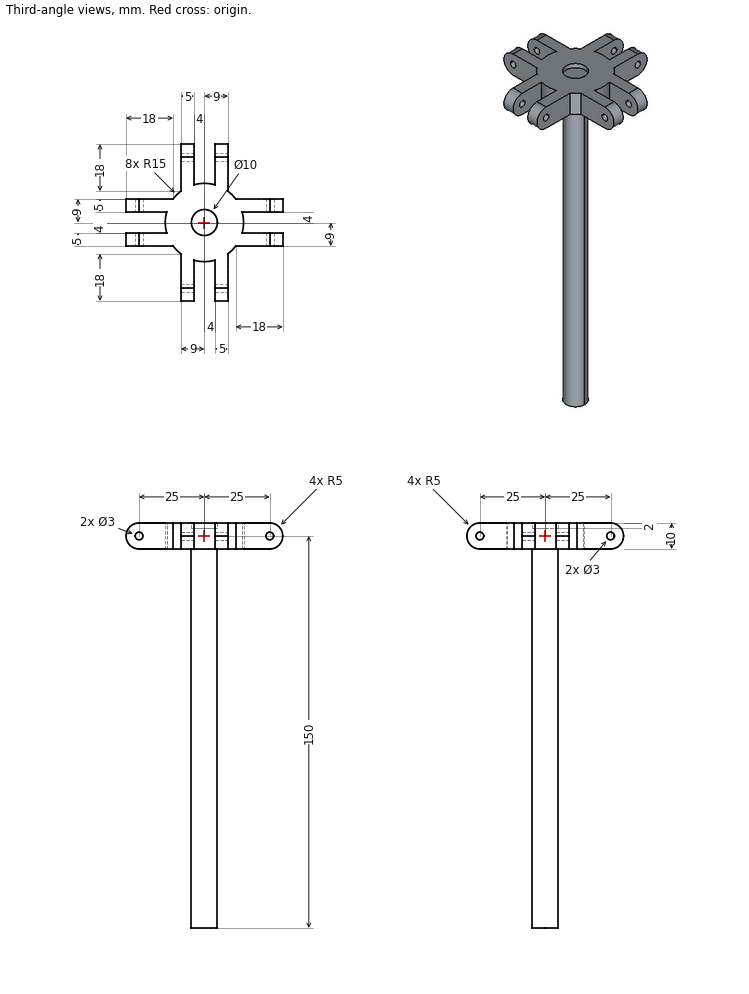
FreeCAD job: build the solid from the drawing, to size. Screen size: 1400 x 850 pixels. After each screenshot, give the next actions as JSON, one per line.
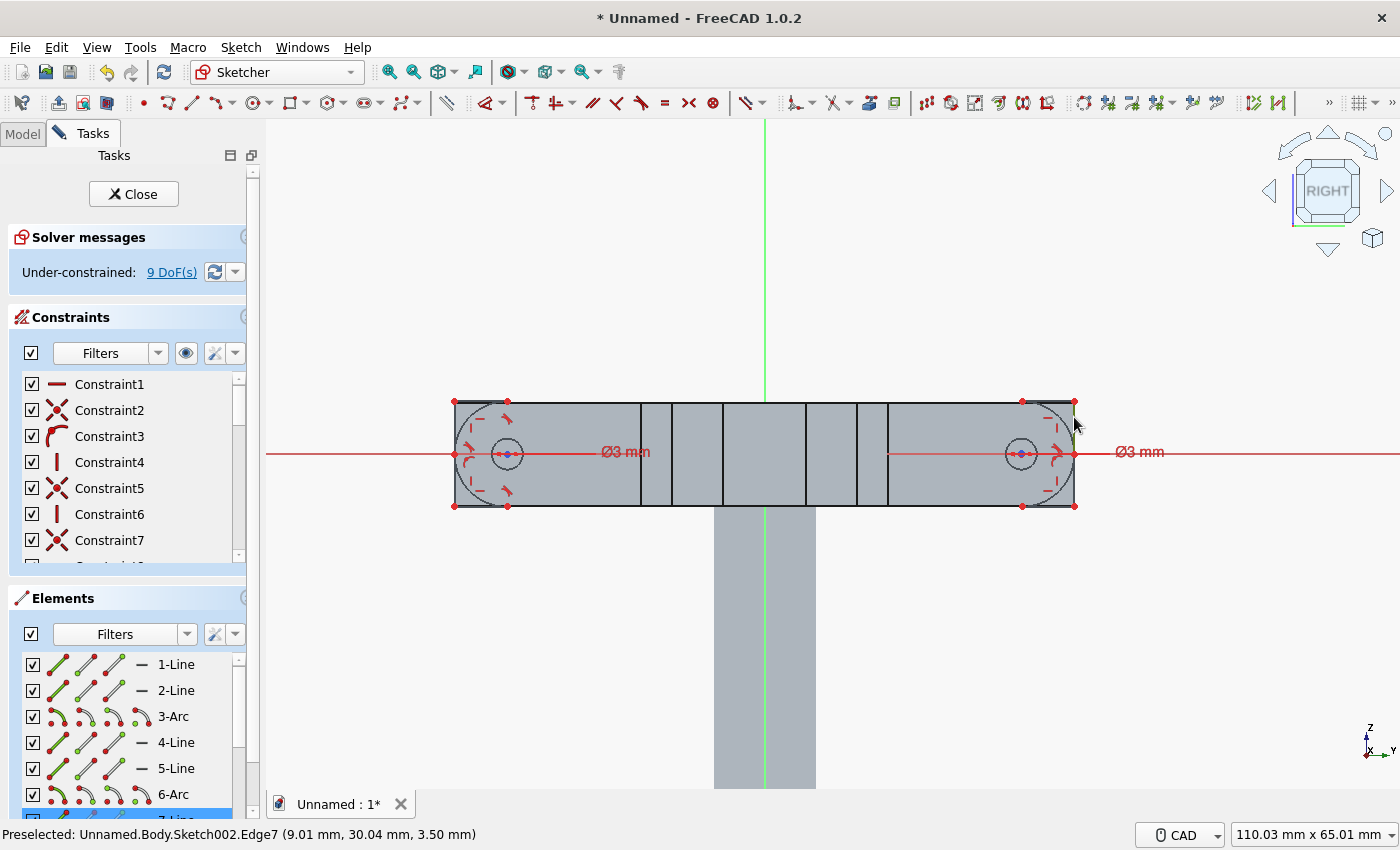
{"action": "left_click", "coordinate": [1059, 491]}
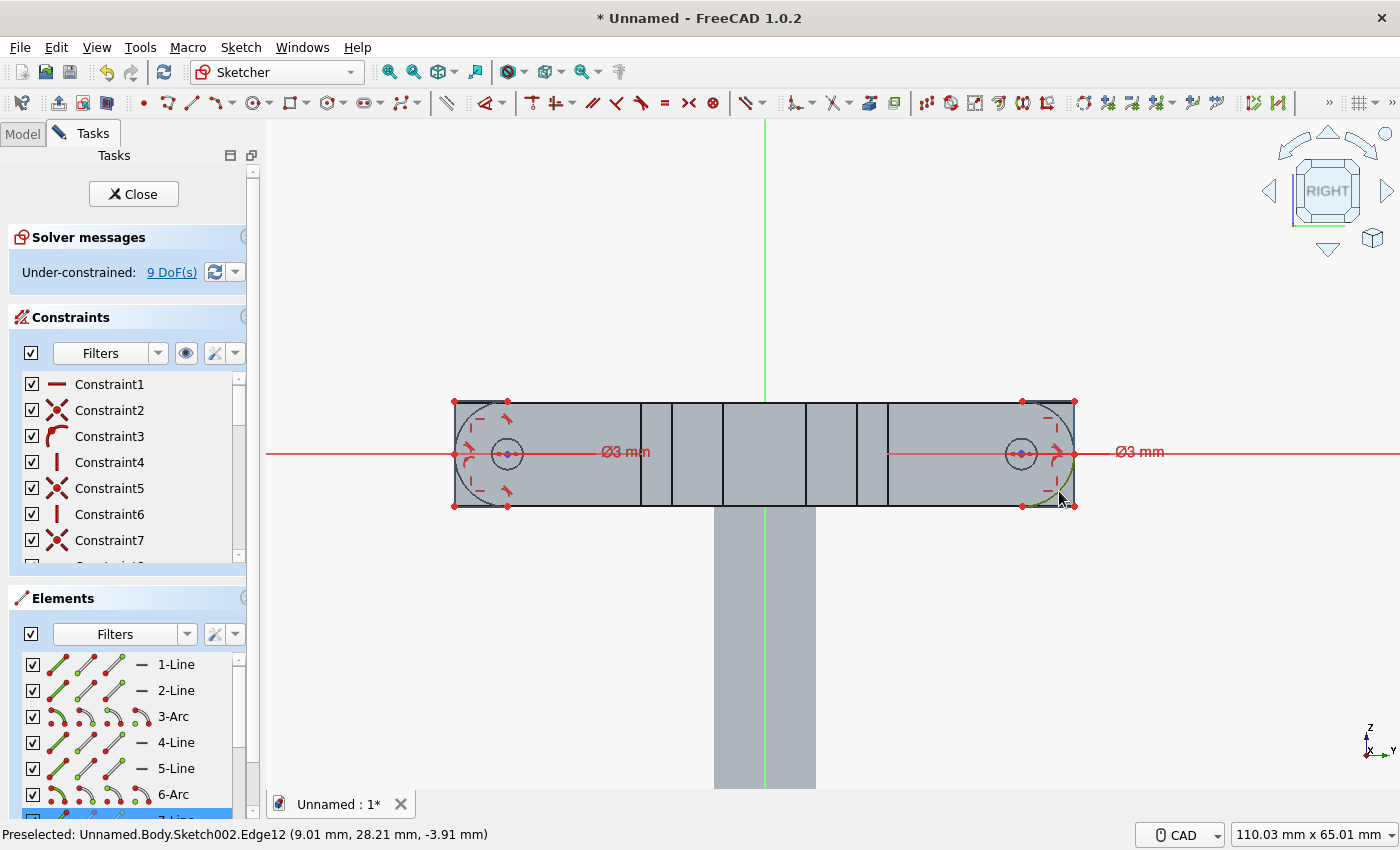
{"action": "left_click", "coordinate": [642, 104]}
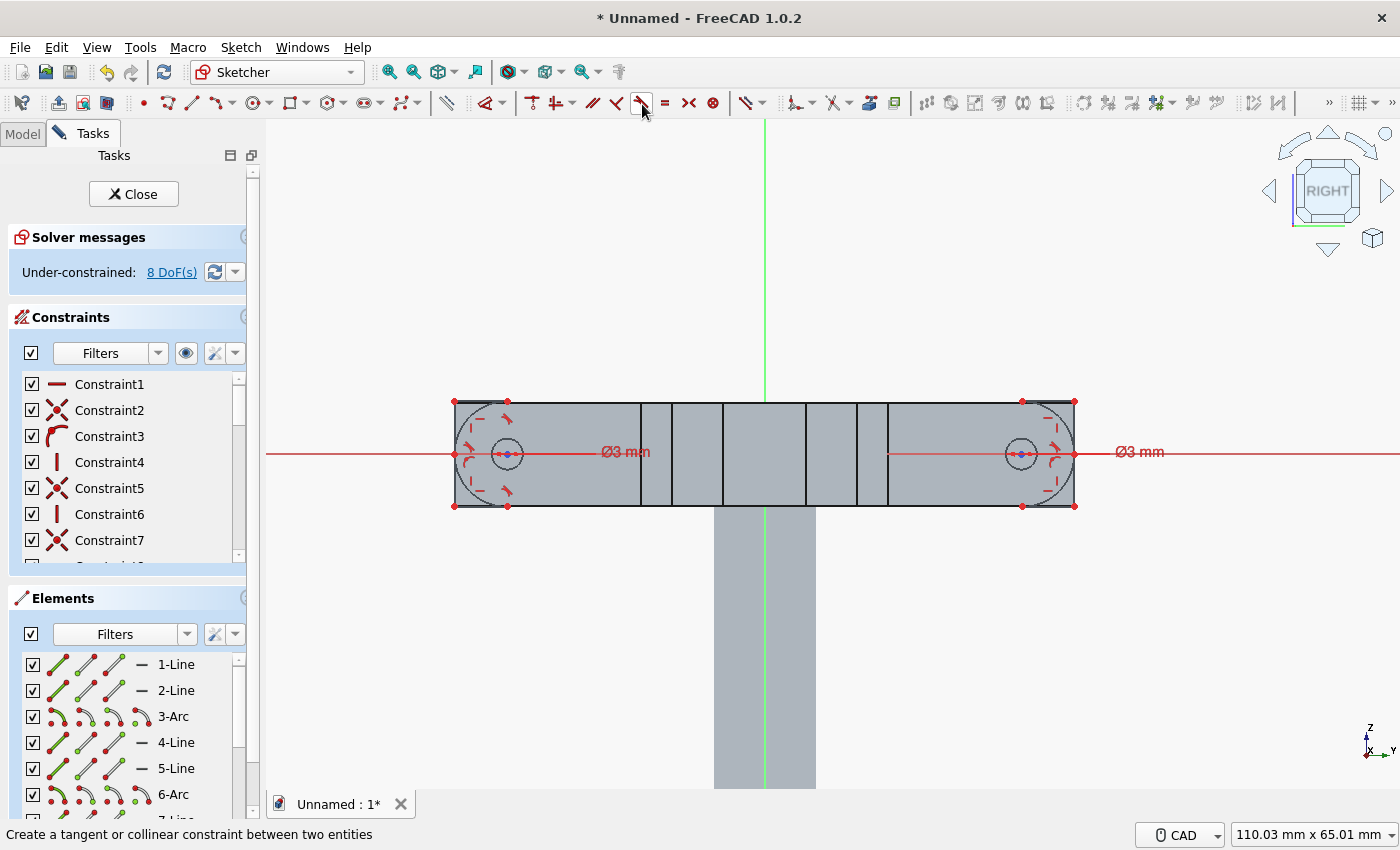
{"action": "left_click", "coordinate": [1059, 401]}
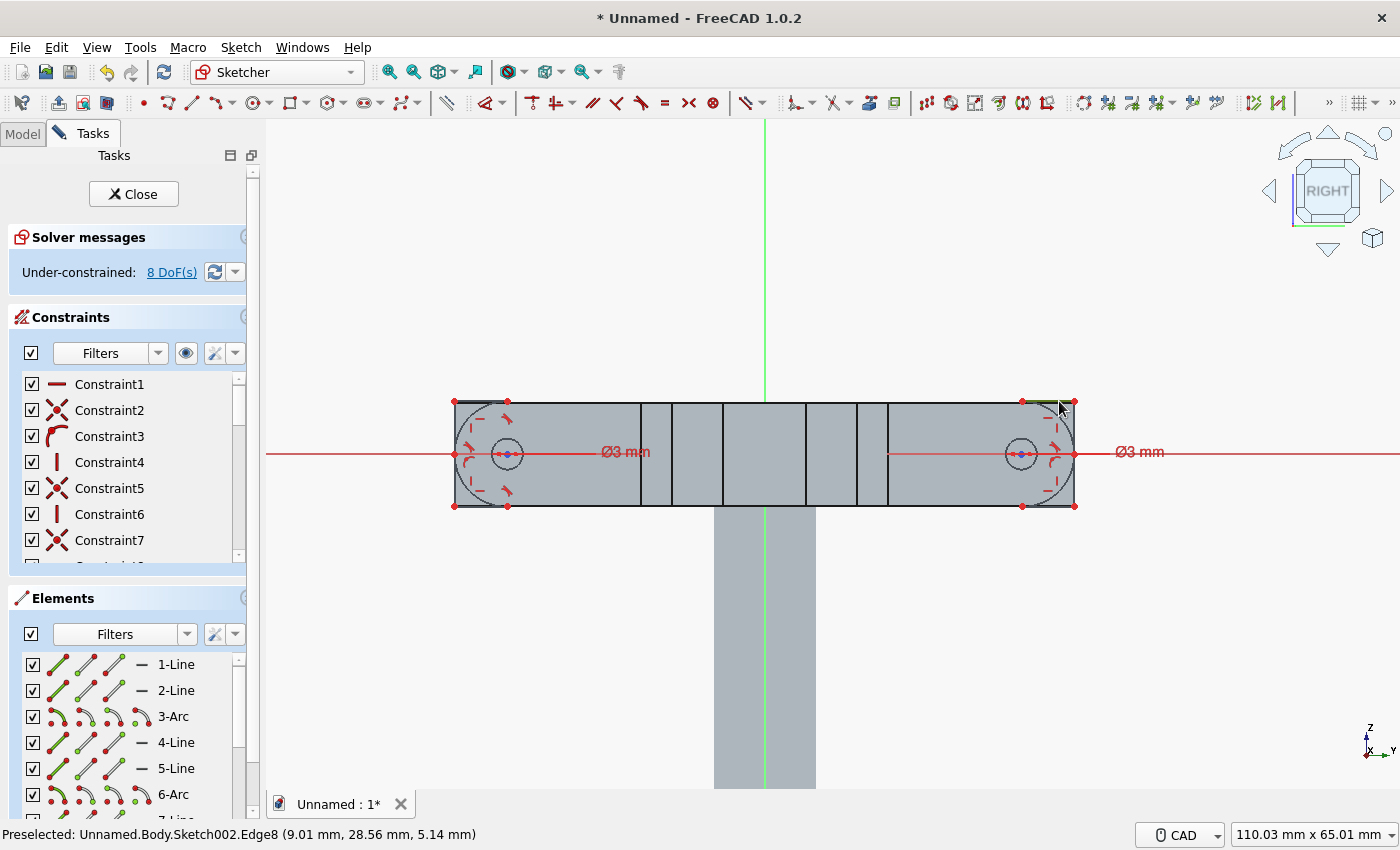
{"action": "left_click", "coordinate": [1059, 417]}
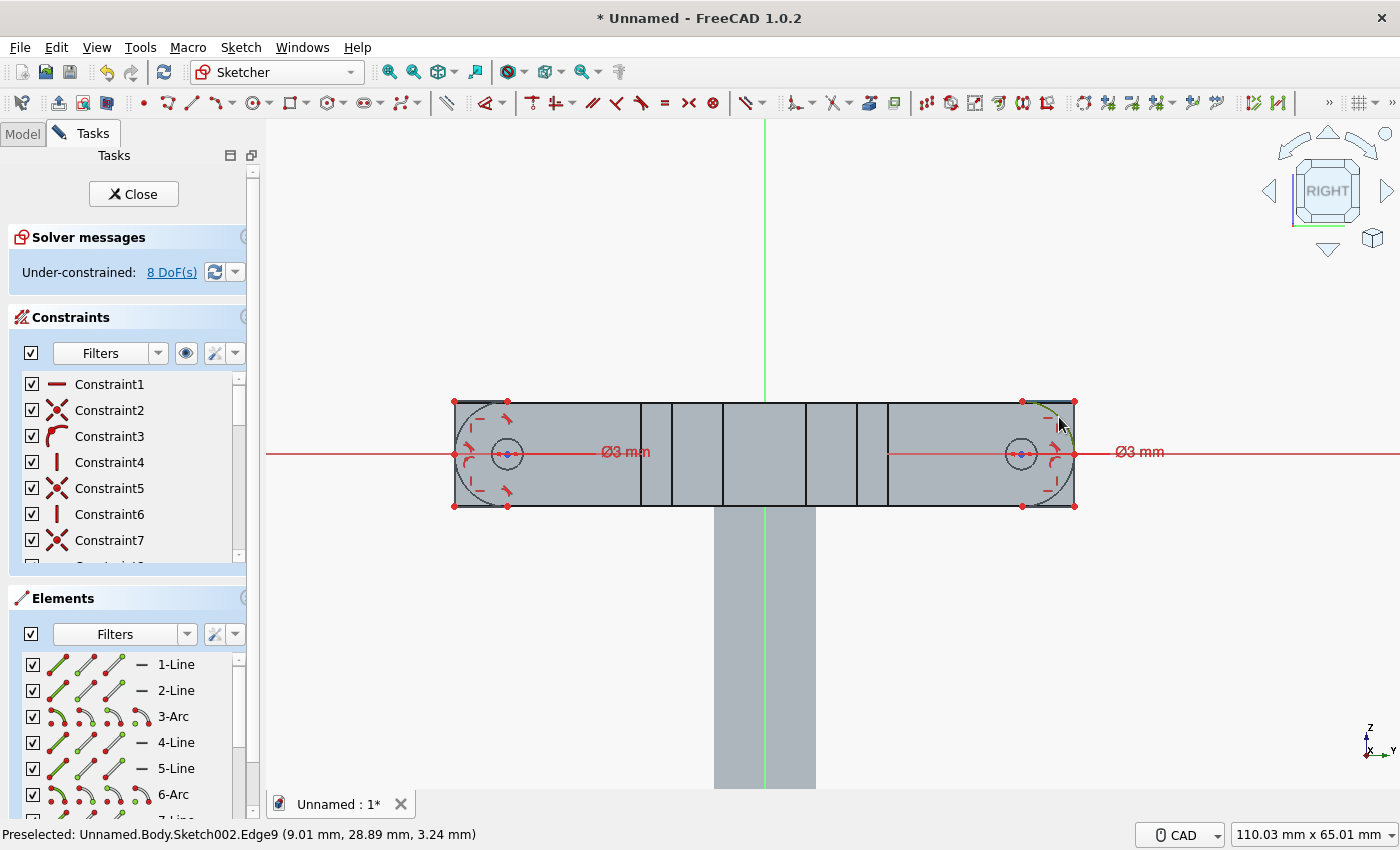
{"action": "key", "text": "t"}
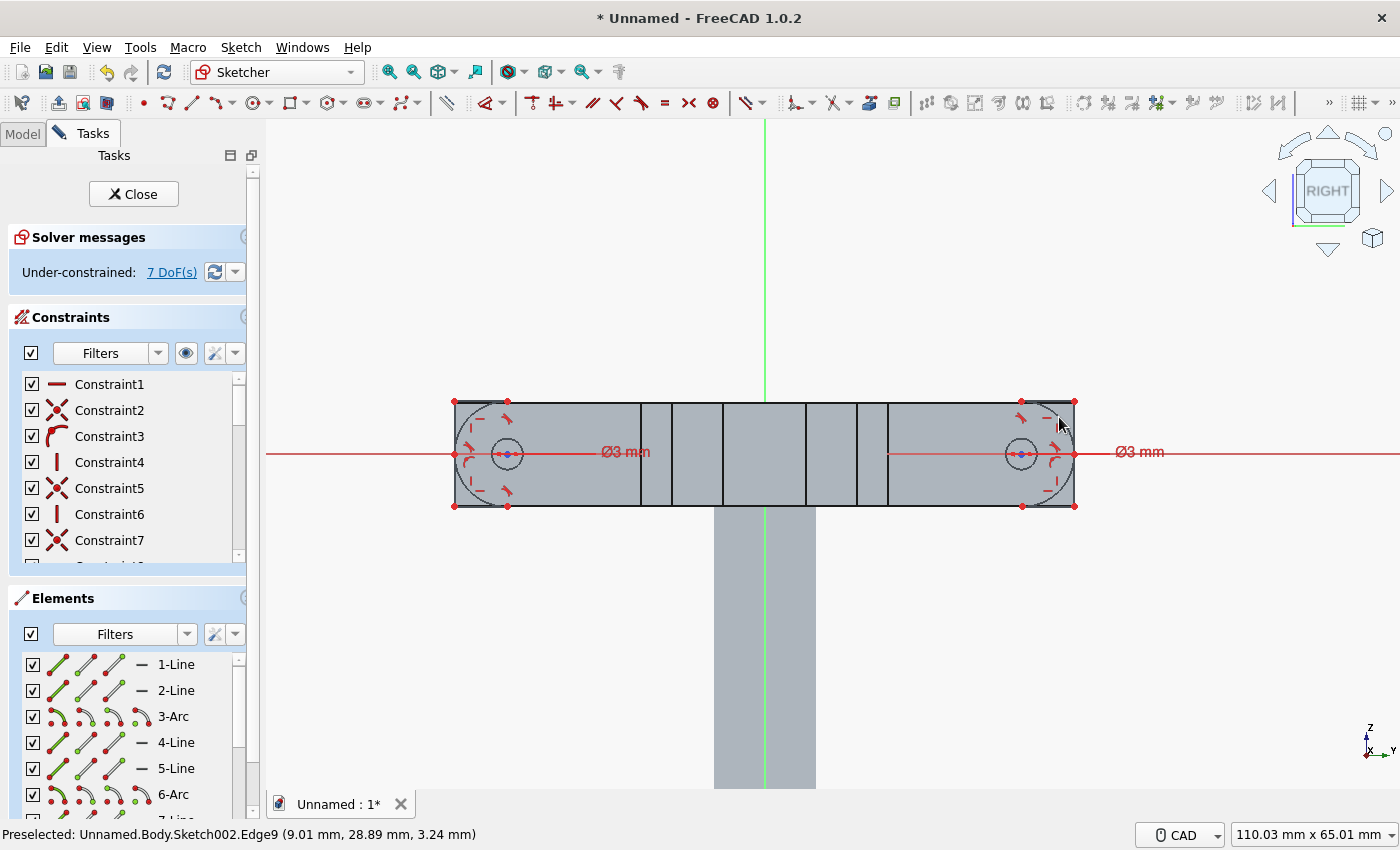
{"action": "left_click", "coordinate": [1059, 507]}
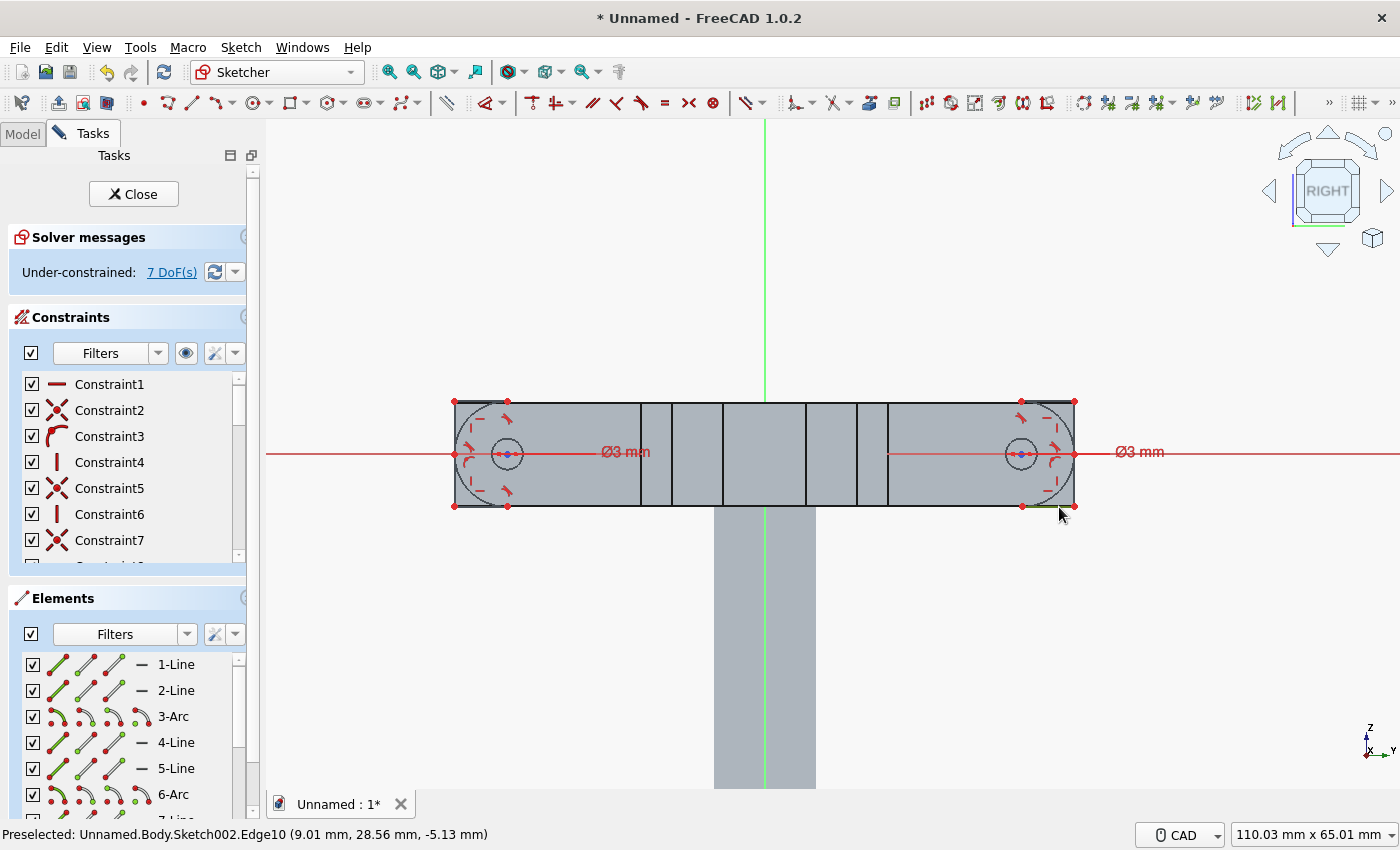
{"action": "left_click", "coordinate": [1059, 491]}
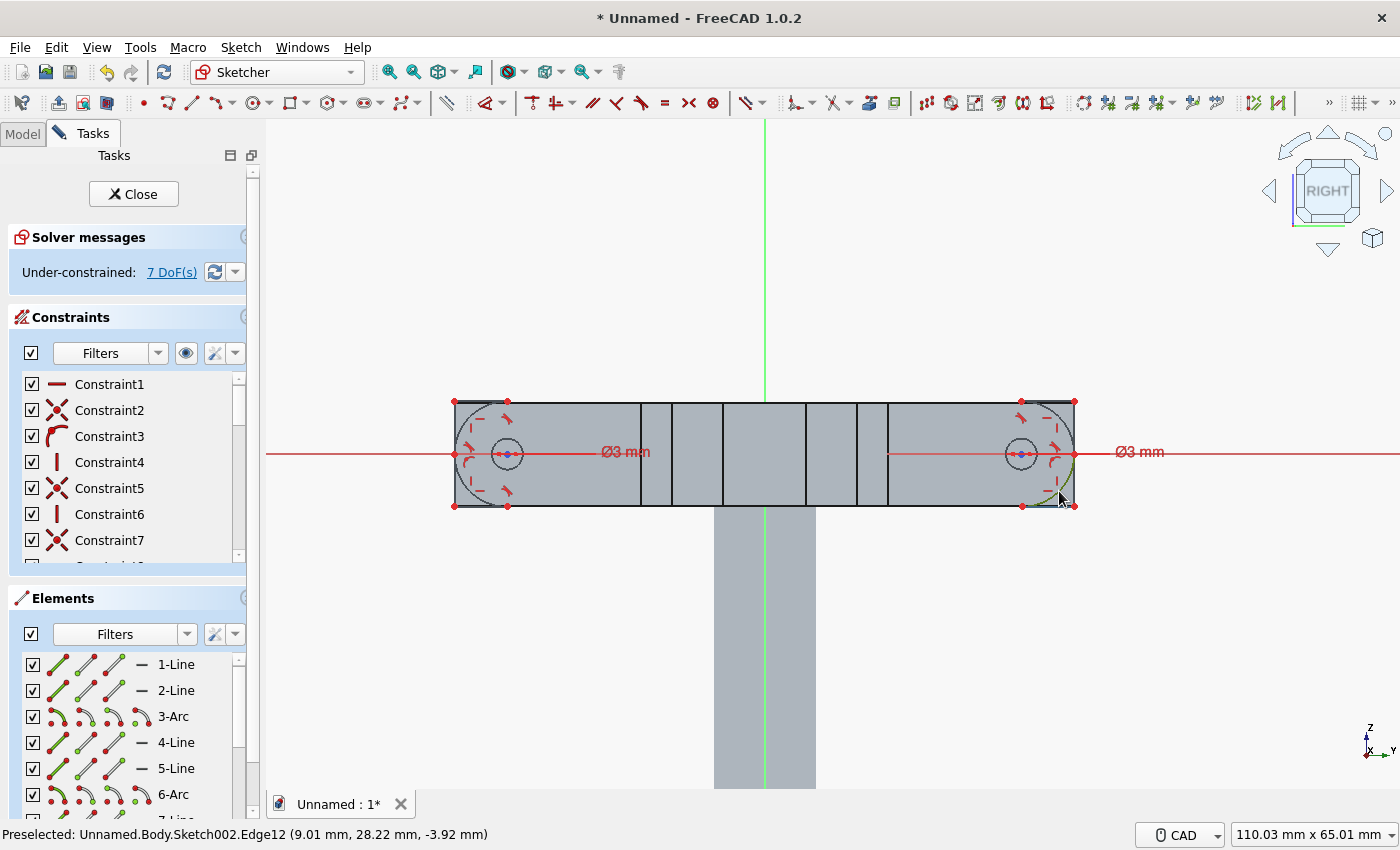
{"action": "left_click", "coordinate": [642, 104]}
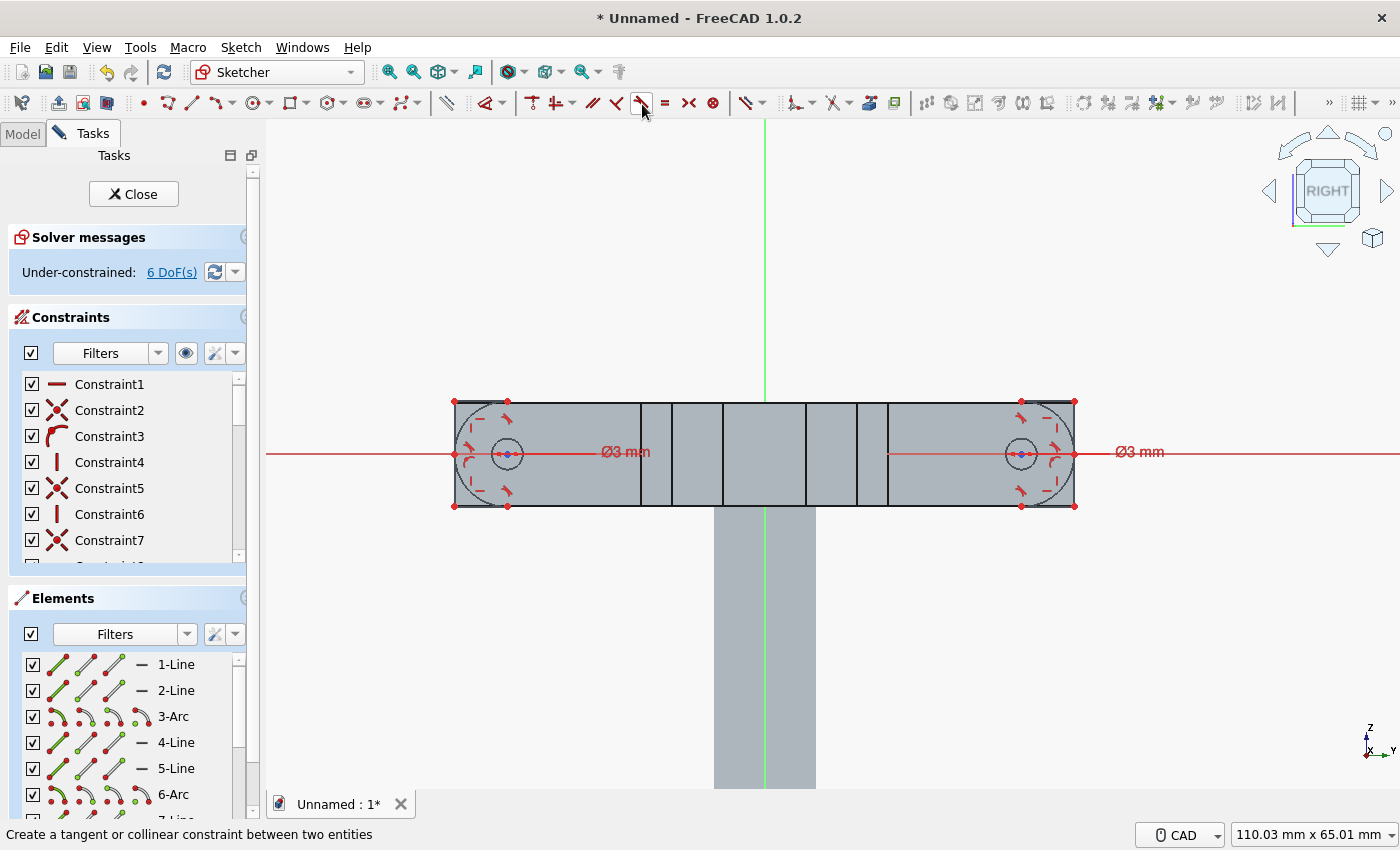
{"action": "left_click", "coordinate": [470, 417]}